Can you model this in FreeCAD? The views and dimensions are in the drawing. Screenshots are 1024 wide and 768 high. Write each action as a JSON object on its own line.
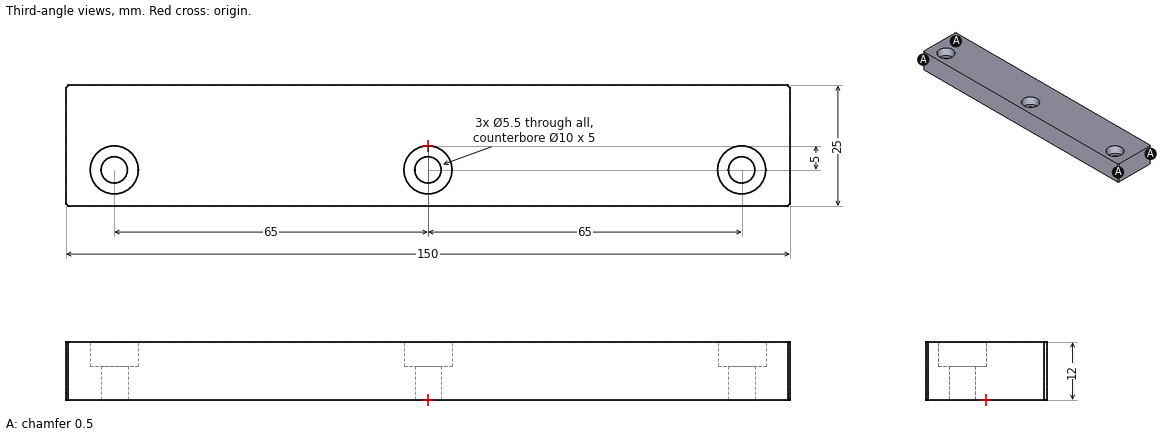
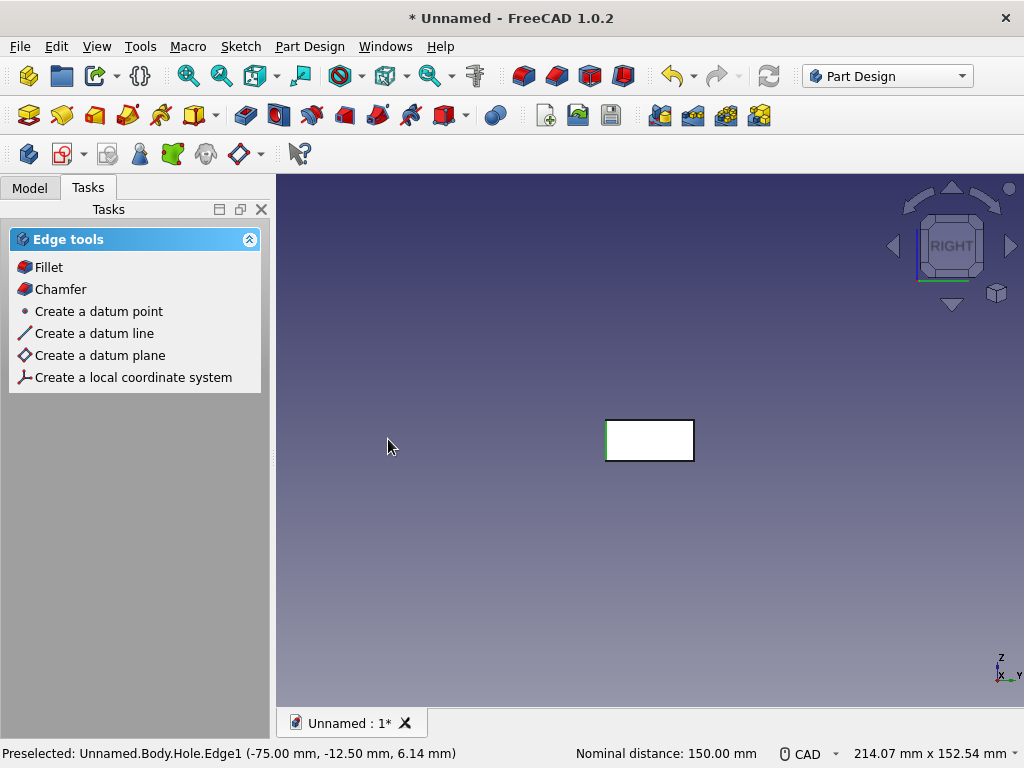
{"action": "left_click", "coordinate": [189, 76]}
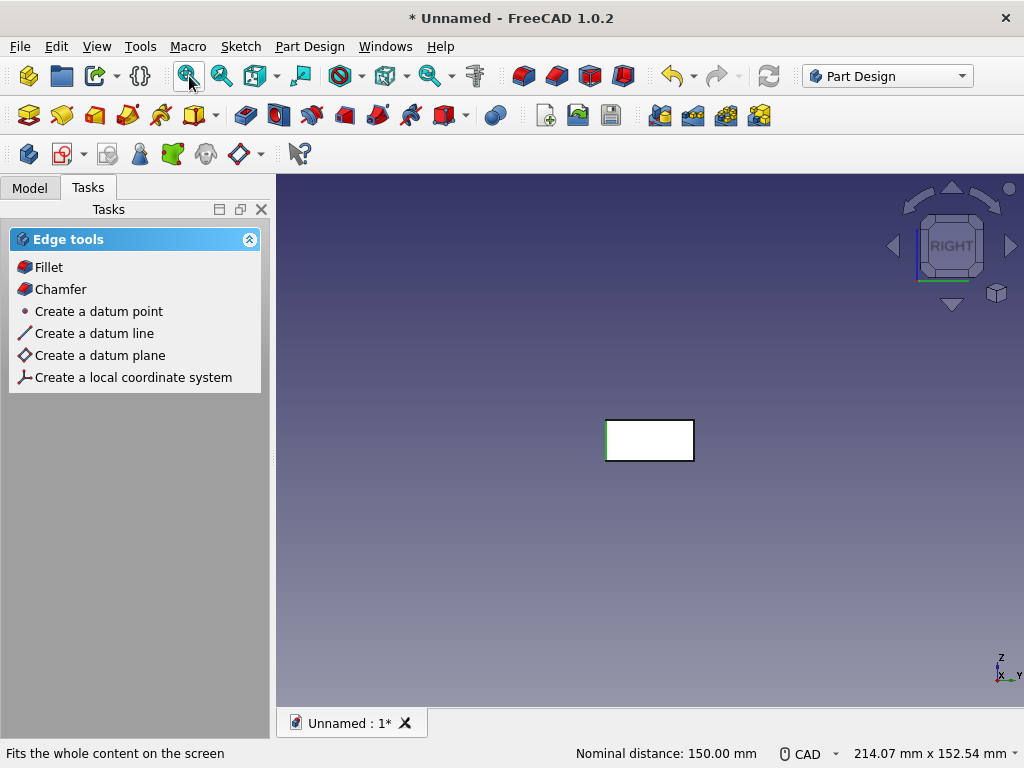
{"action": "left_click", "coordinate": [694, 439], "text": "ctrl"}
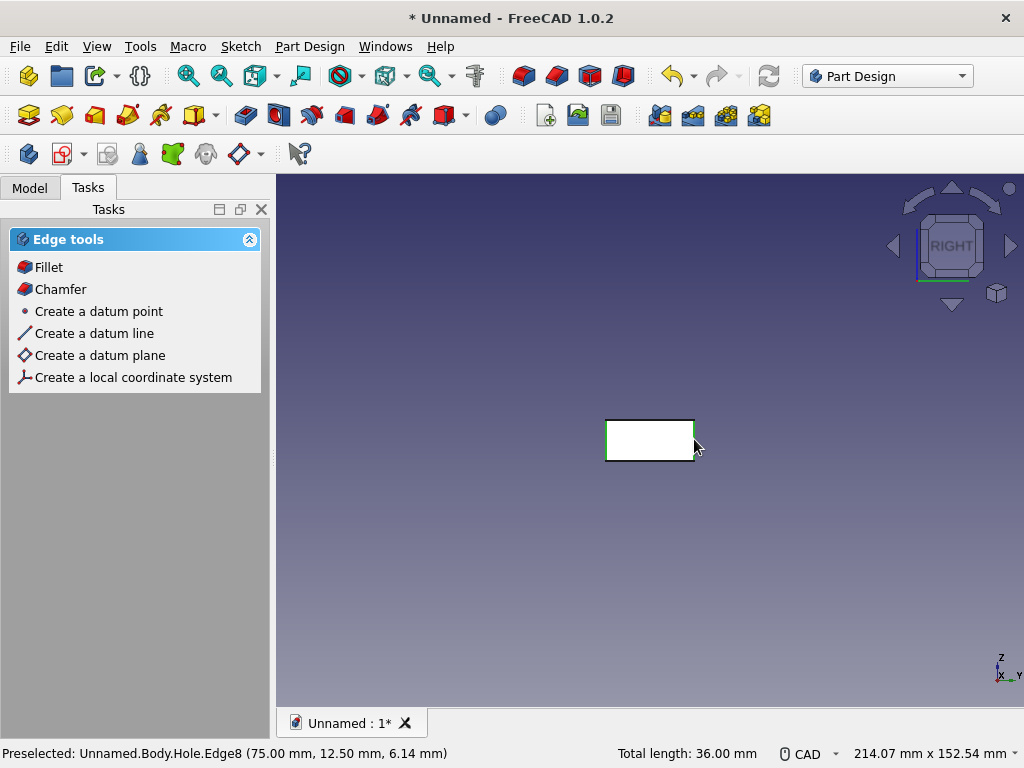
{"action": "key", "text": "5"}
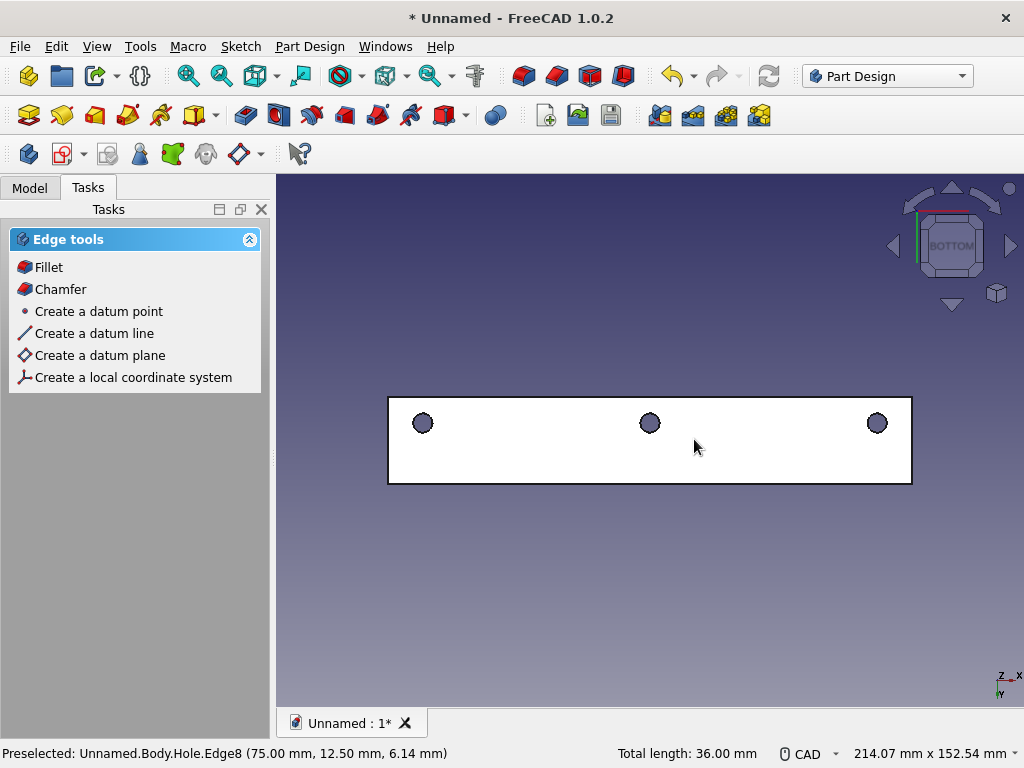
{"action": "key", "text": "4"}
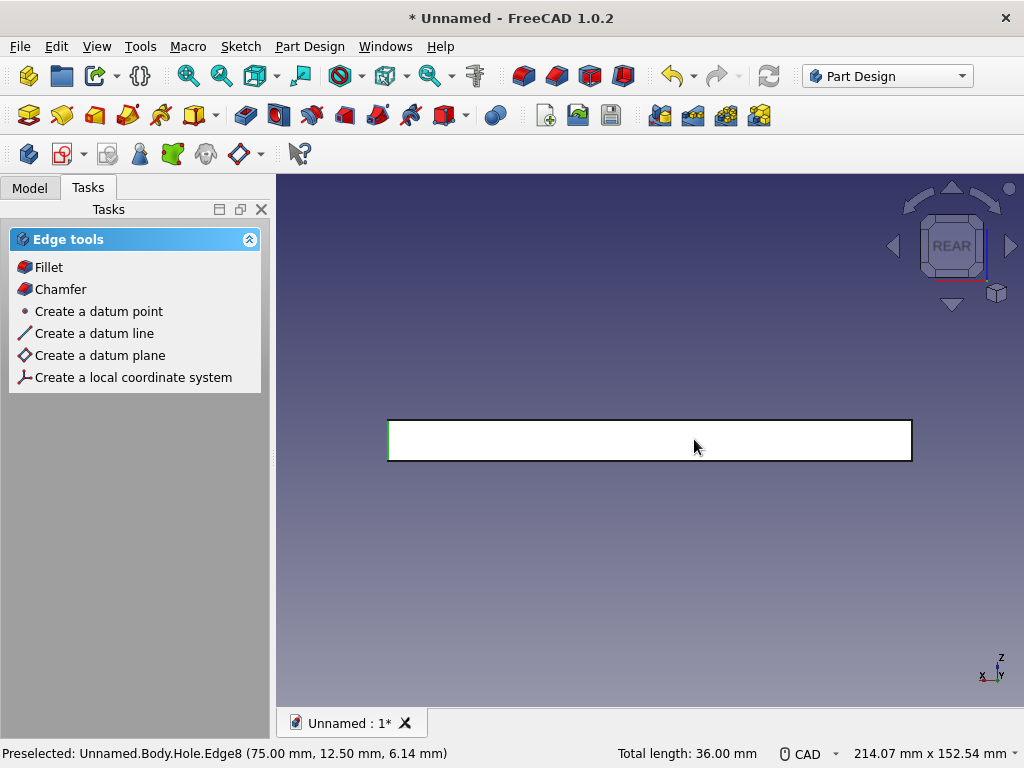
{"action": "left_click", "coordinate": [912, 439], "text": "ctrl"}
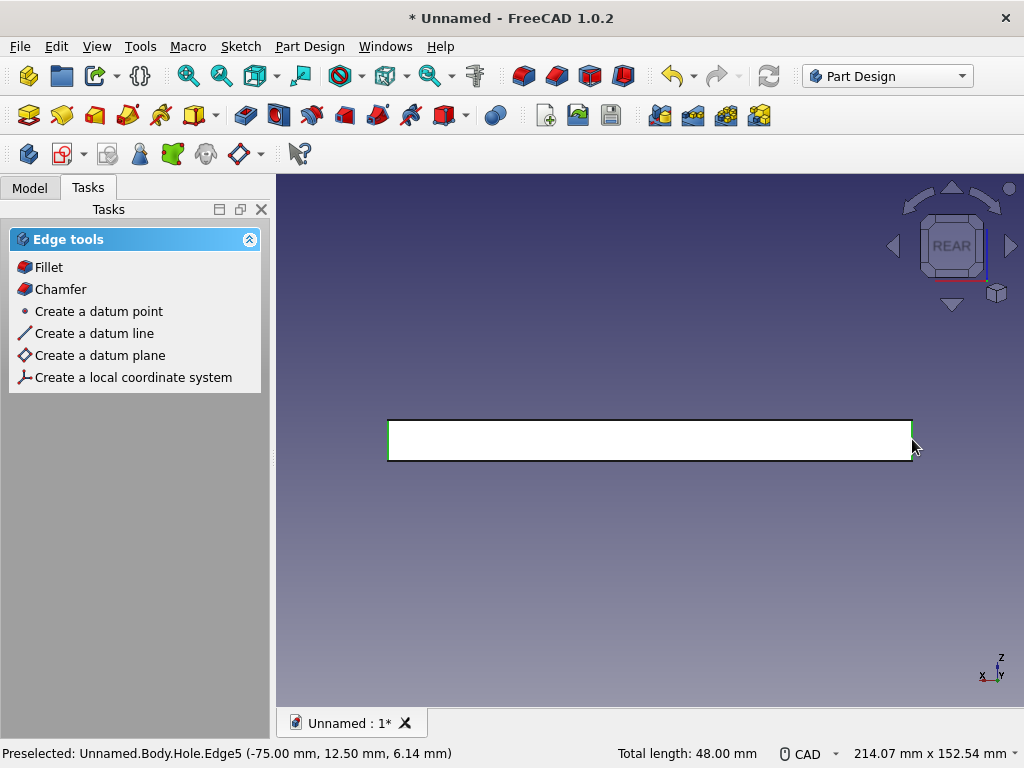
{"action": "left_click", "coordinate": [557, 76]}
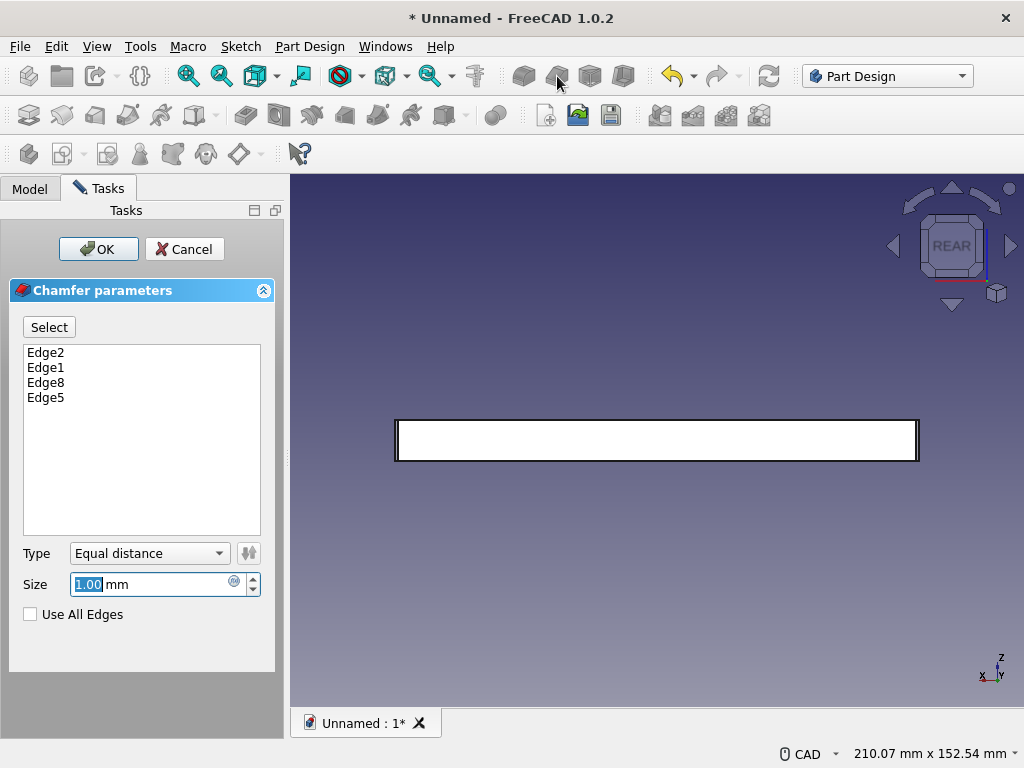
{"action": "type", "text": "0.5"}
{"action": "key", "text": "Tab"}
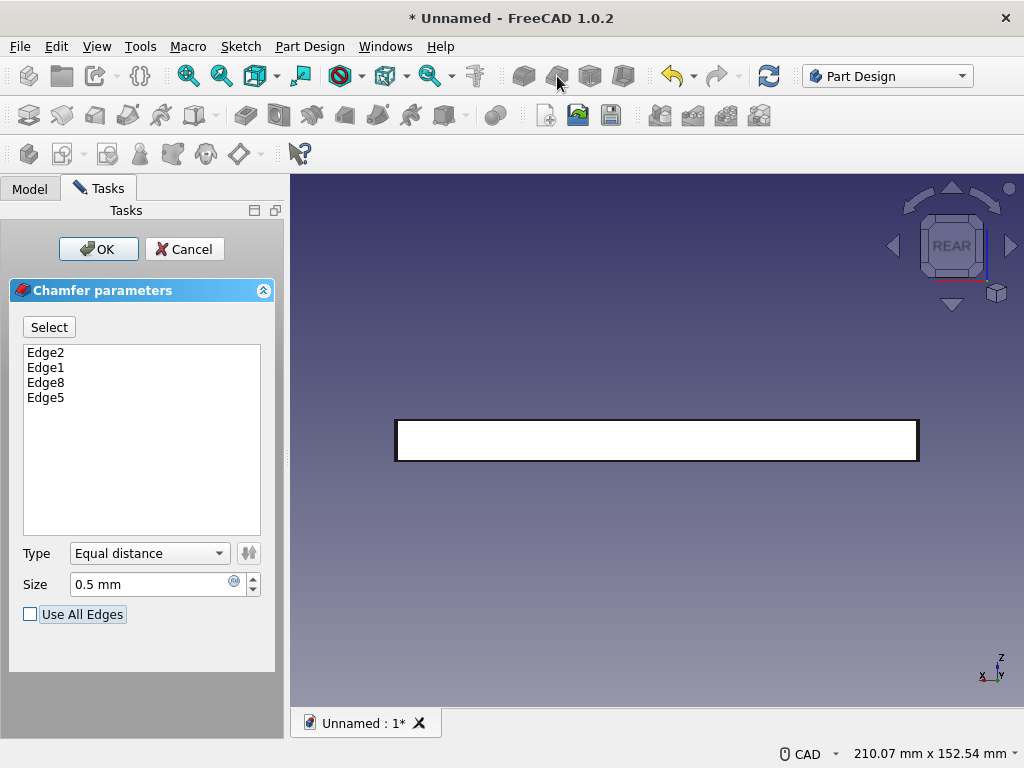
{"action": "left_click", "coordinate": [99, 249]}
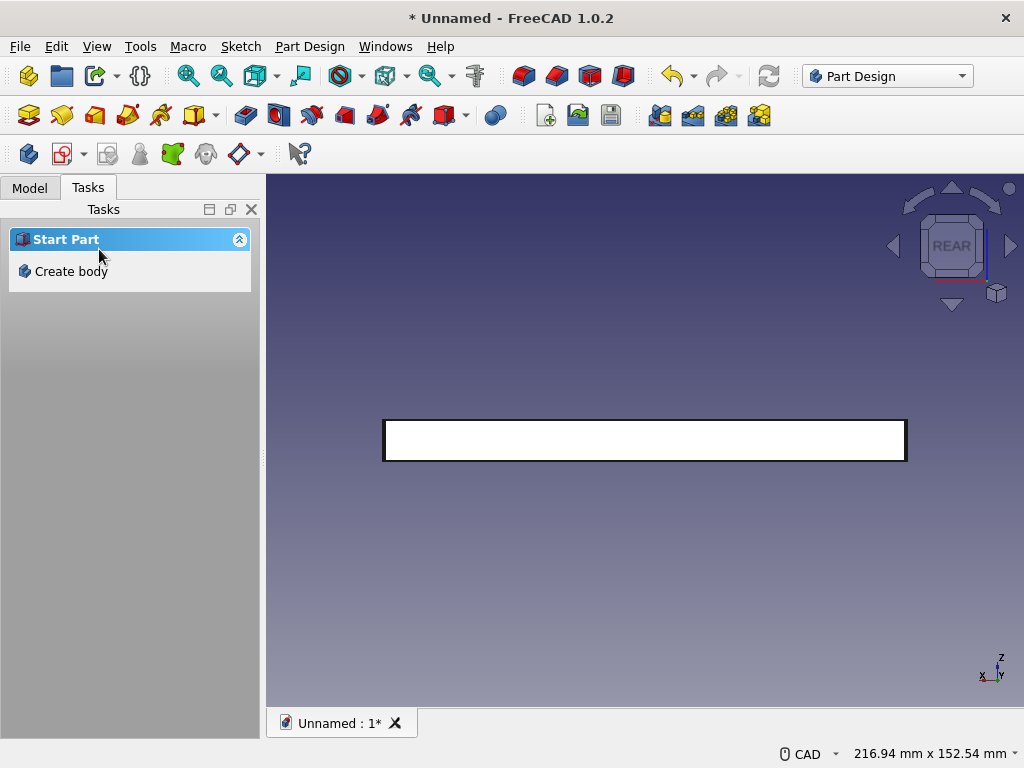
{"action": "key", "text": "0"}